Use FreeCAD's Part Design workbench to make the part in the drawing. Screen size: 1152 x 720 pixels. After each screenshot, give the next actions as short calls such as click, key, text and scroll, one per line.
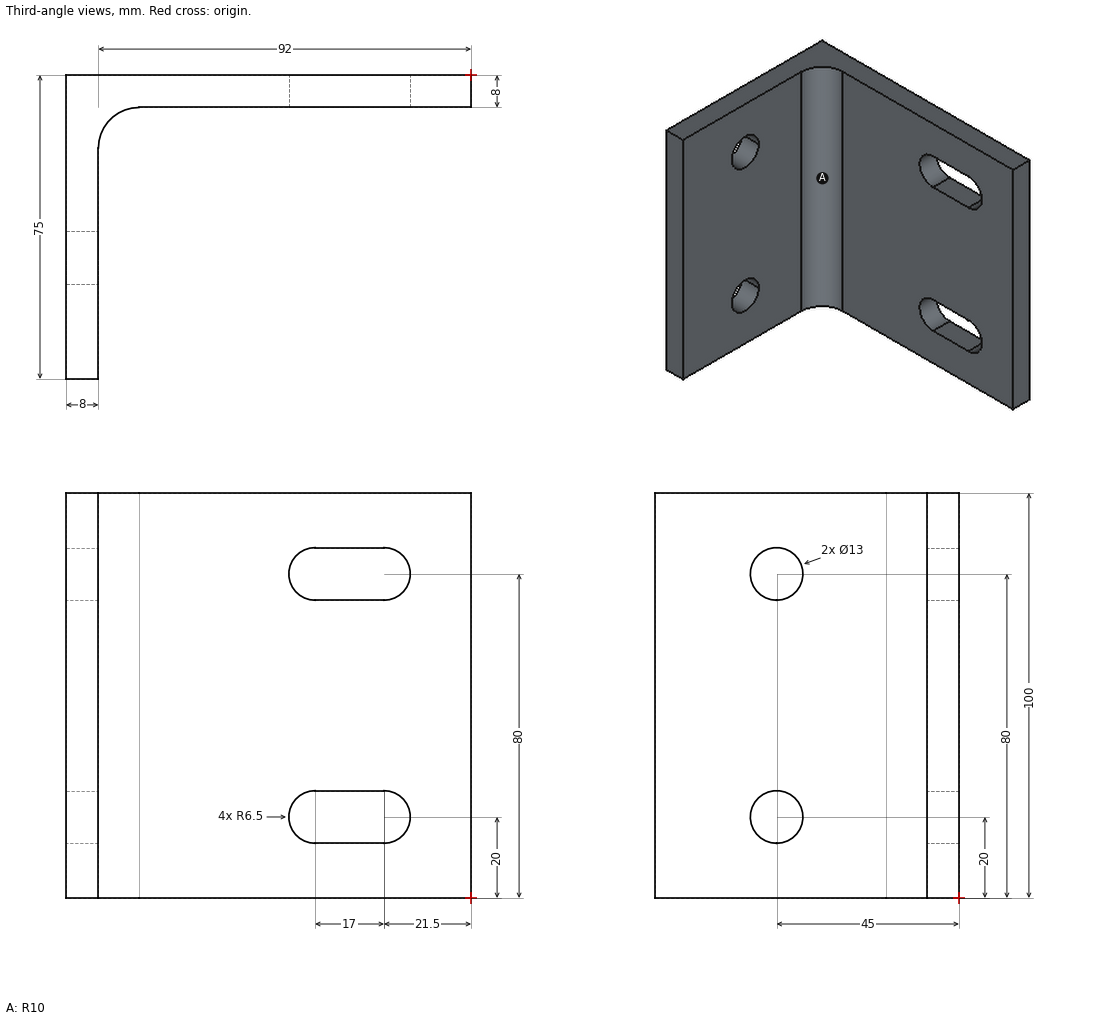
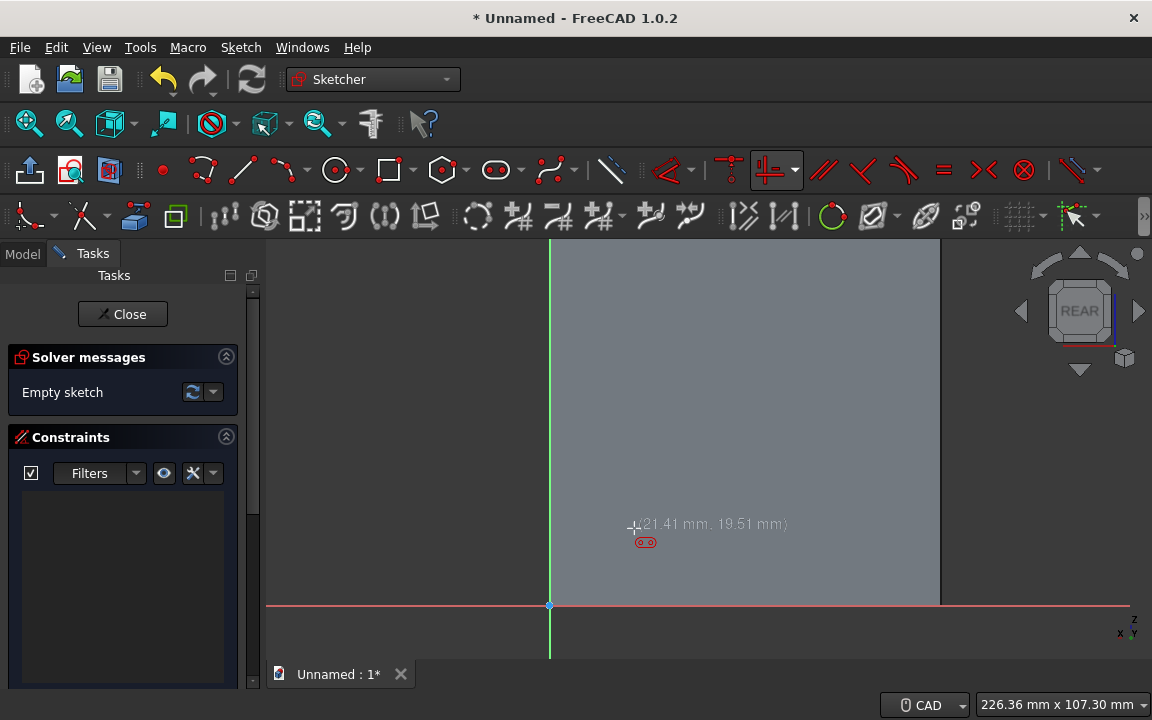
click(634, 527)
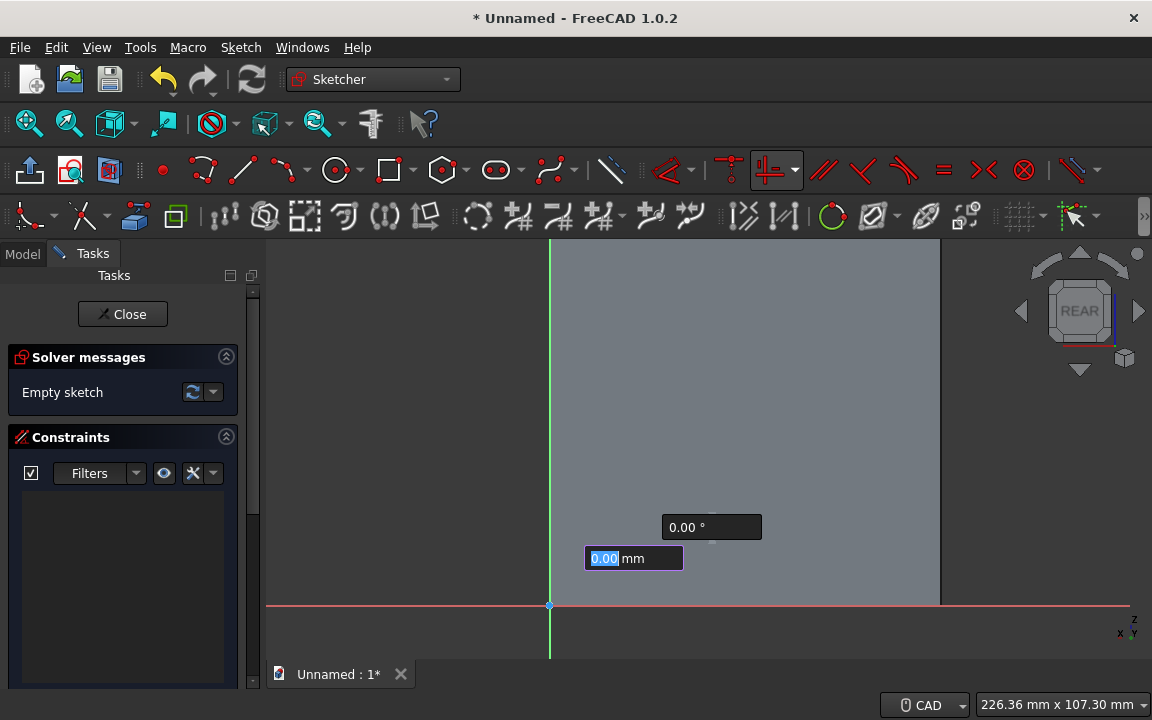
click(701, 527)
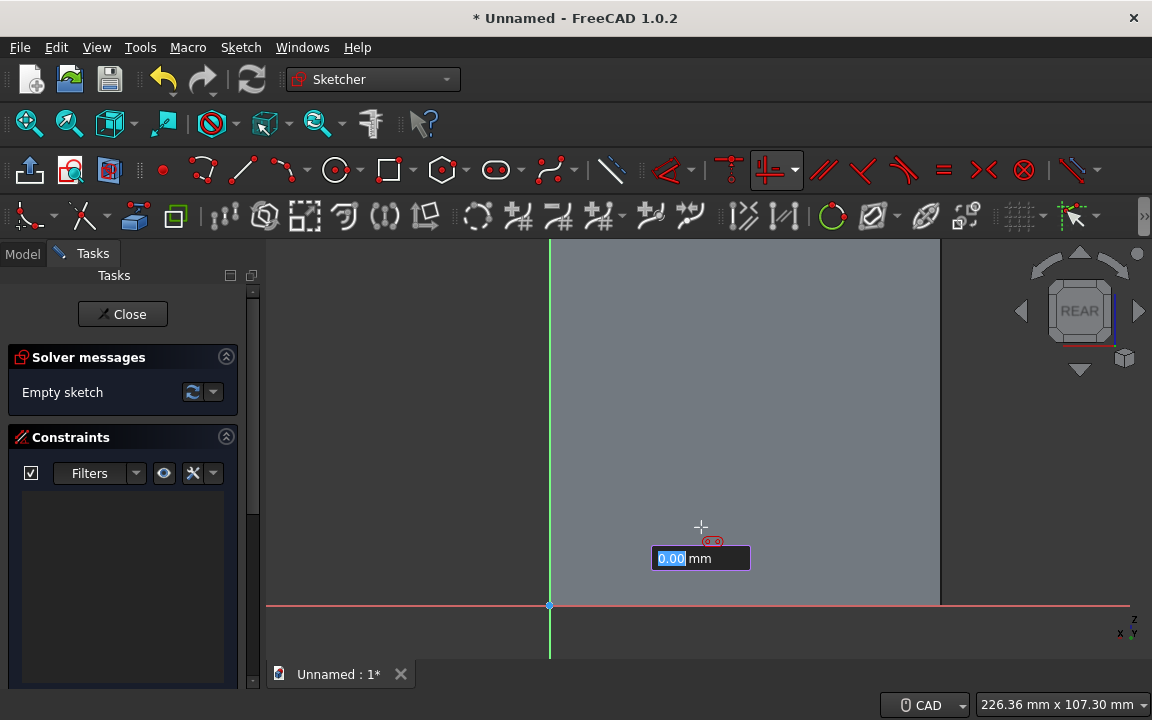
click(667, 553)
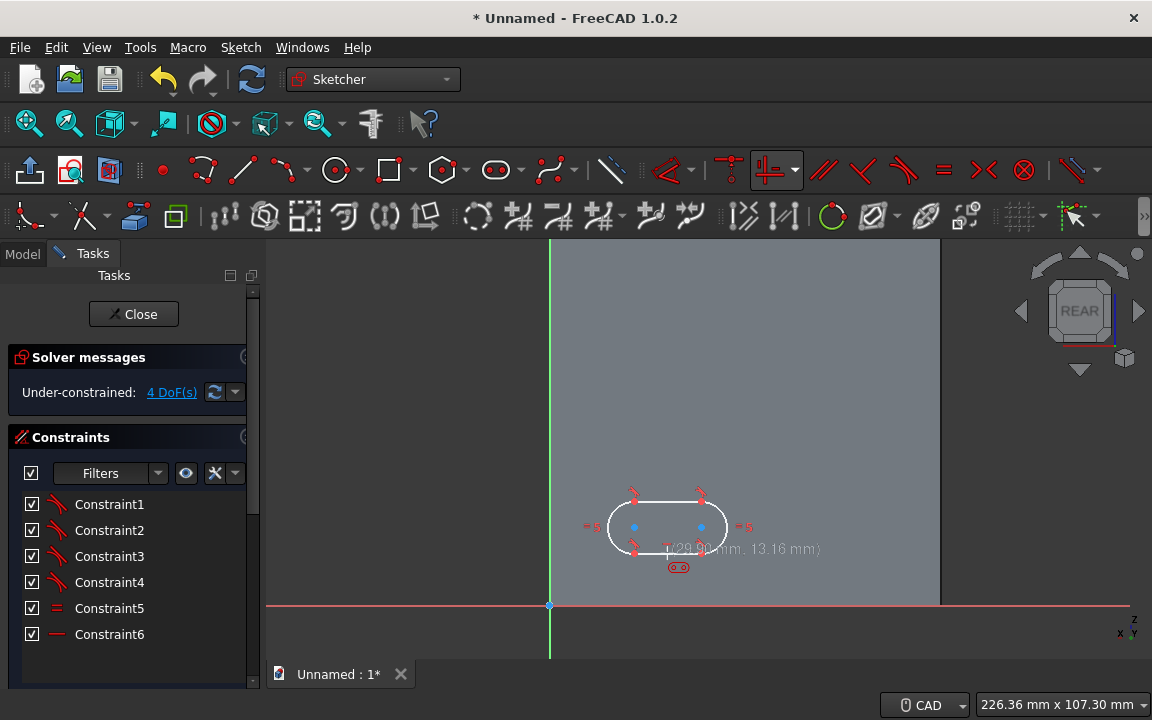
click(634, 292)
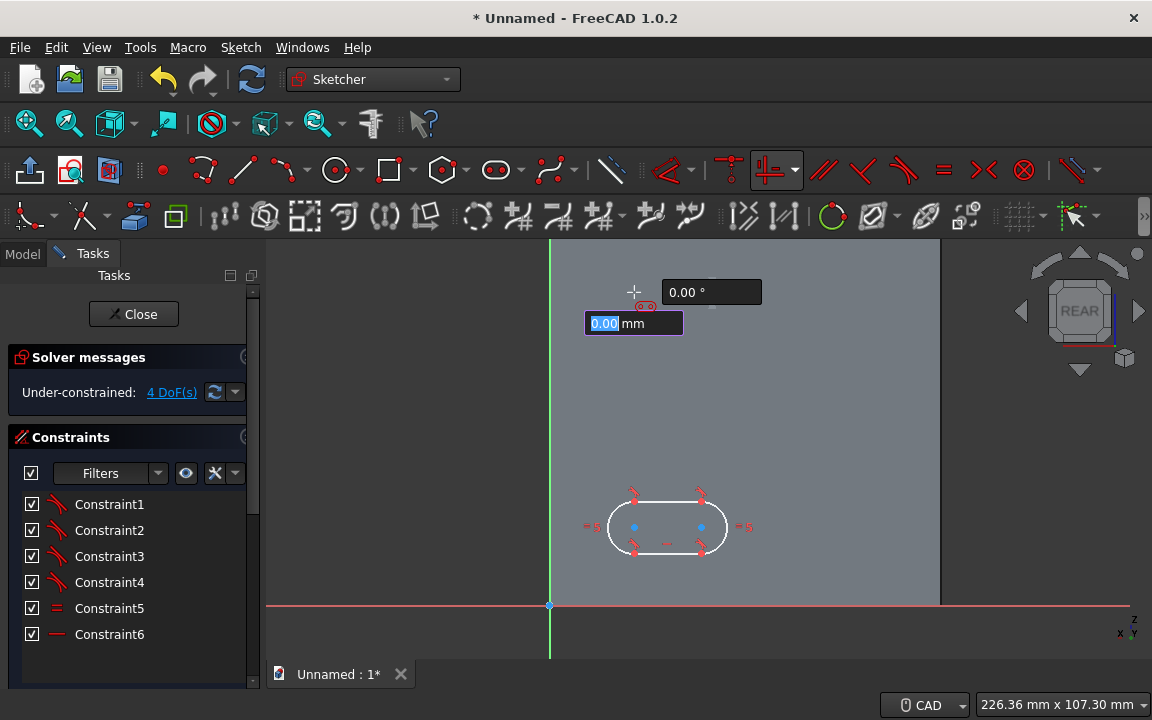
click(701, 292)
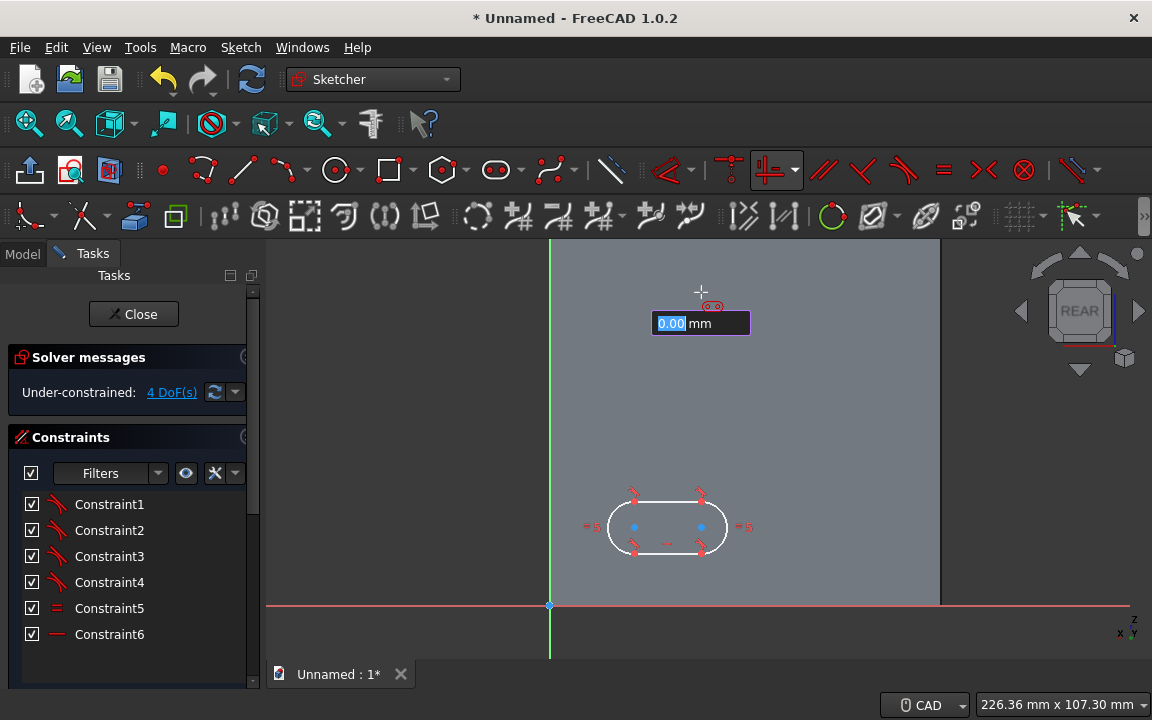
click(667, 318)
key(Escape)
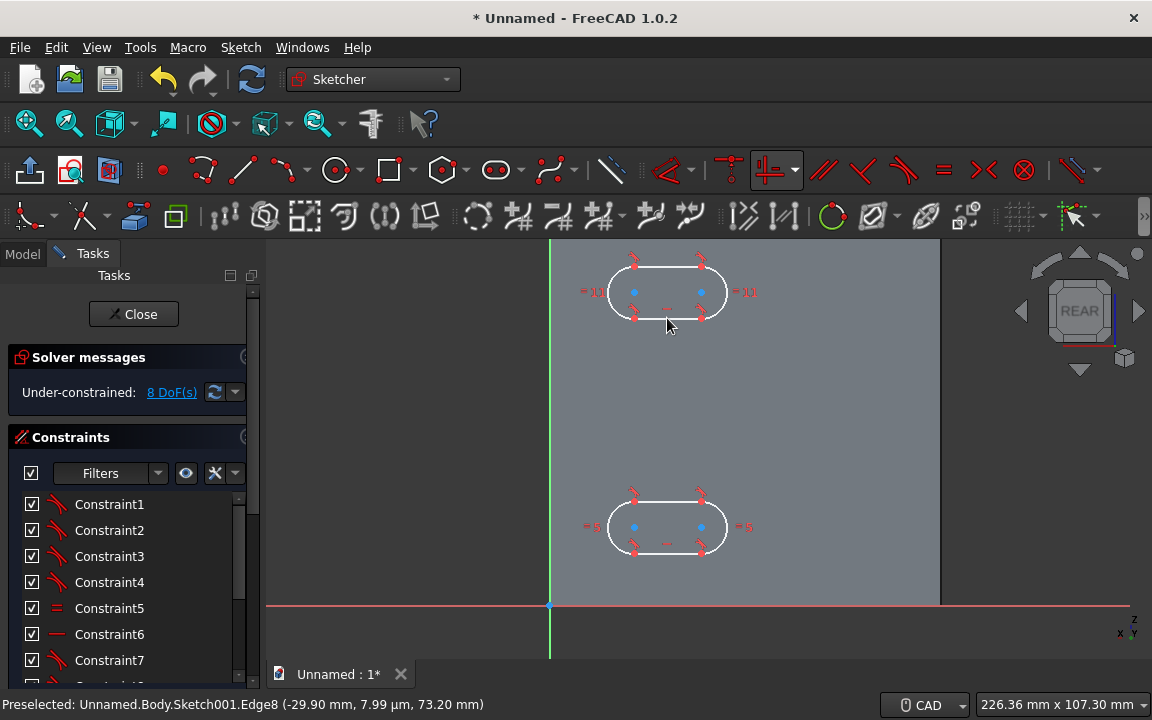
click(613, 513)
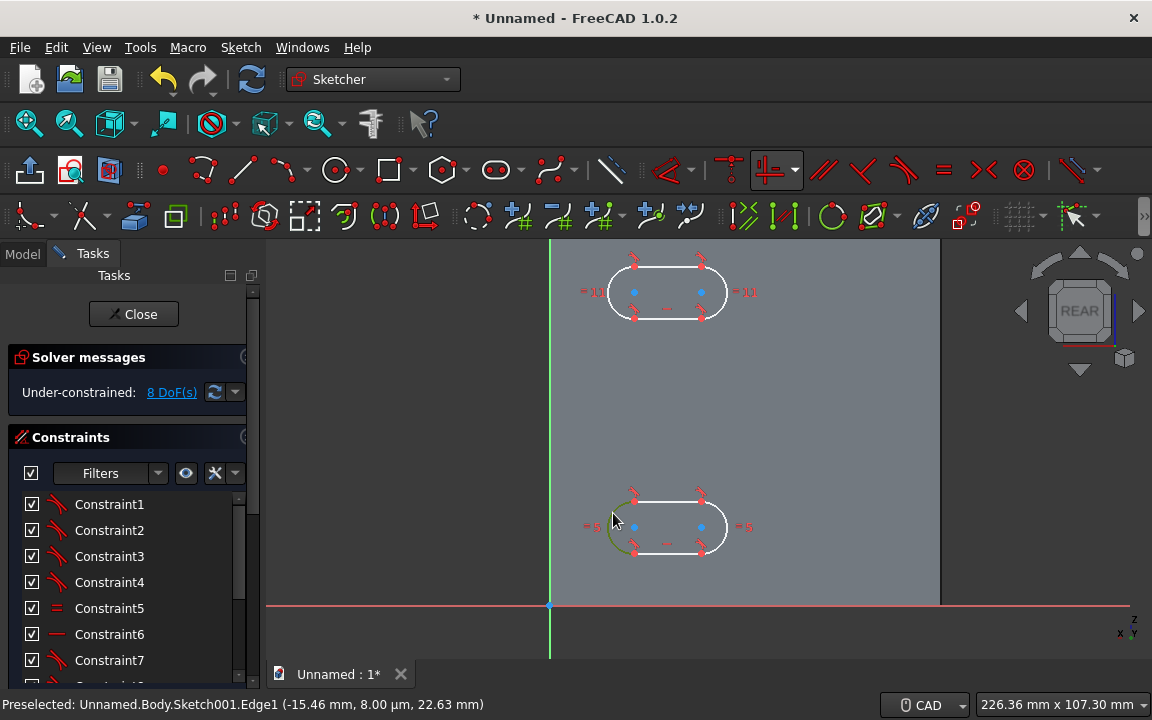
click(613, 278)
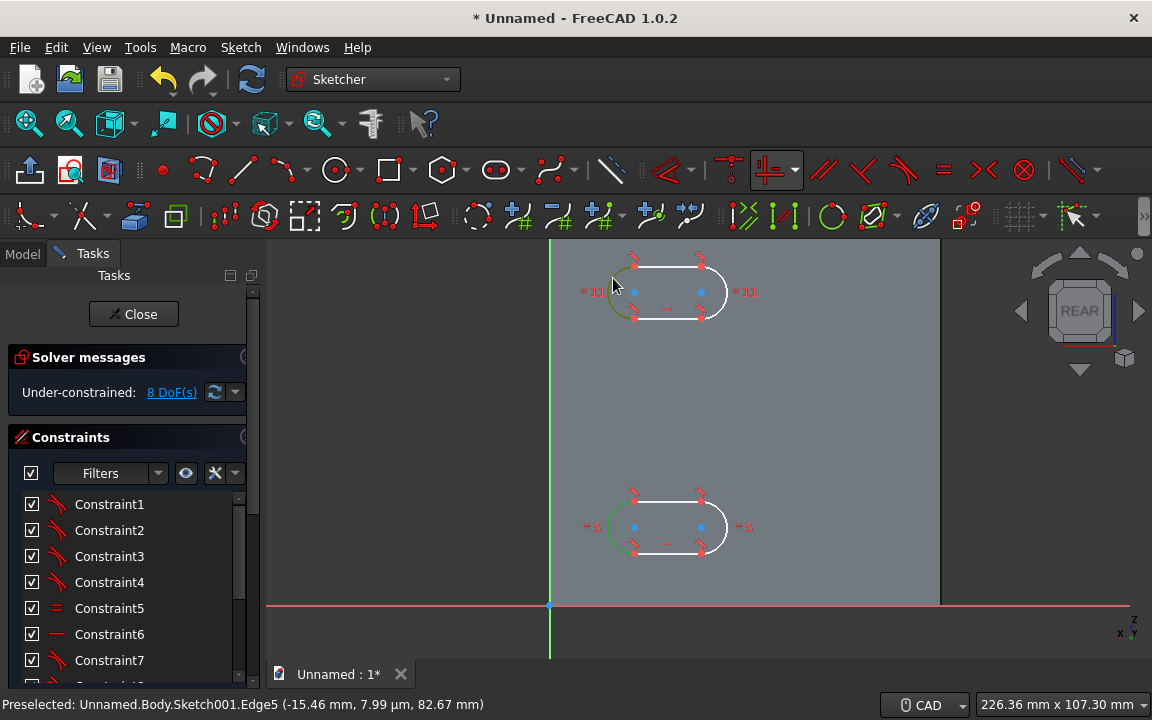
click(944, 170)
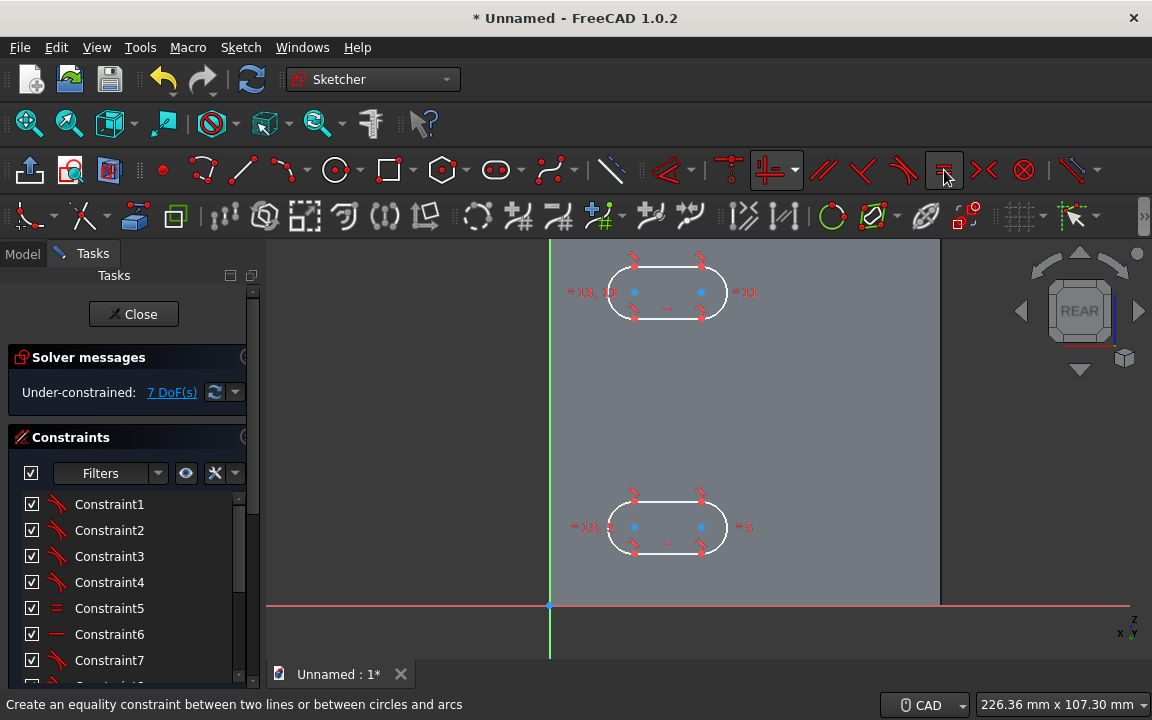
click(666, 170)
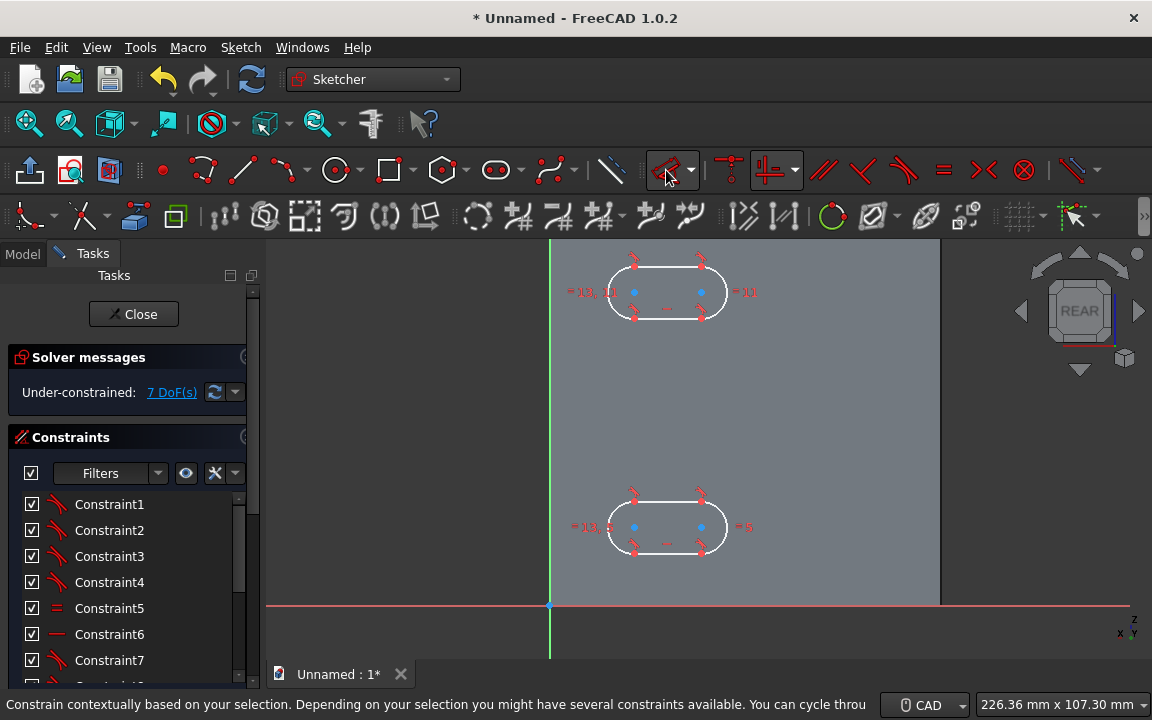
scroll(613, 513, up, 3)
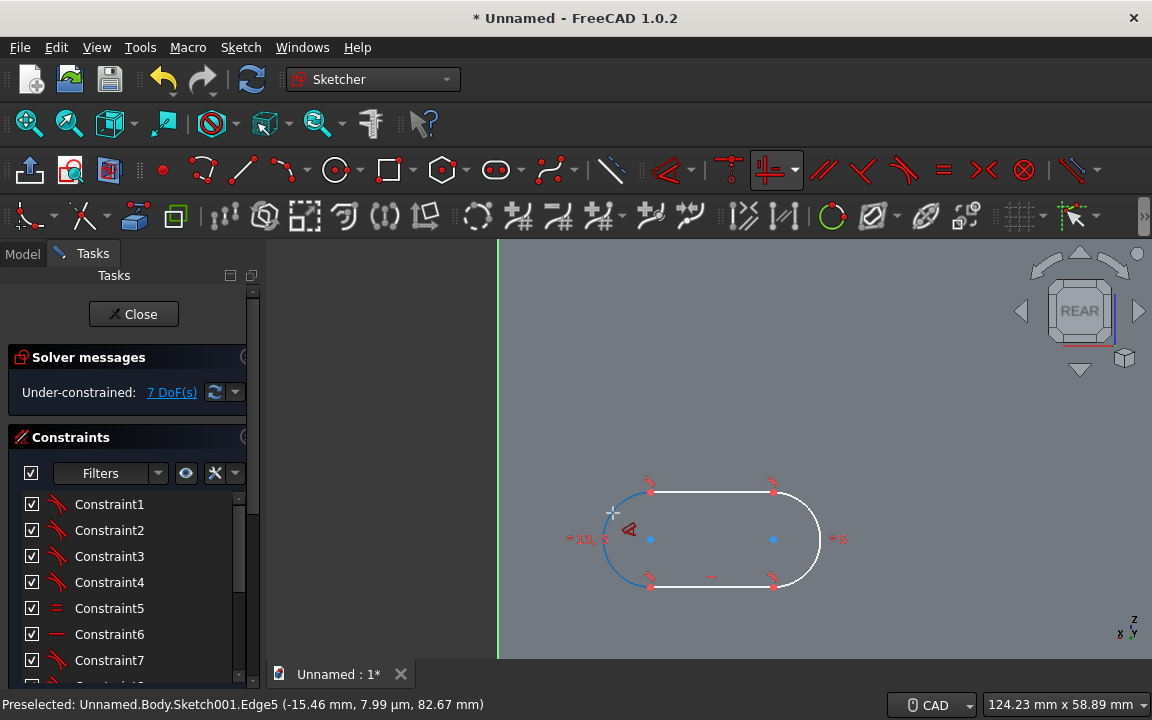
click(613, 512)
click(587, 493)